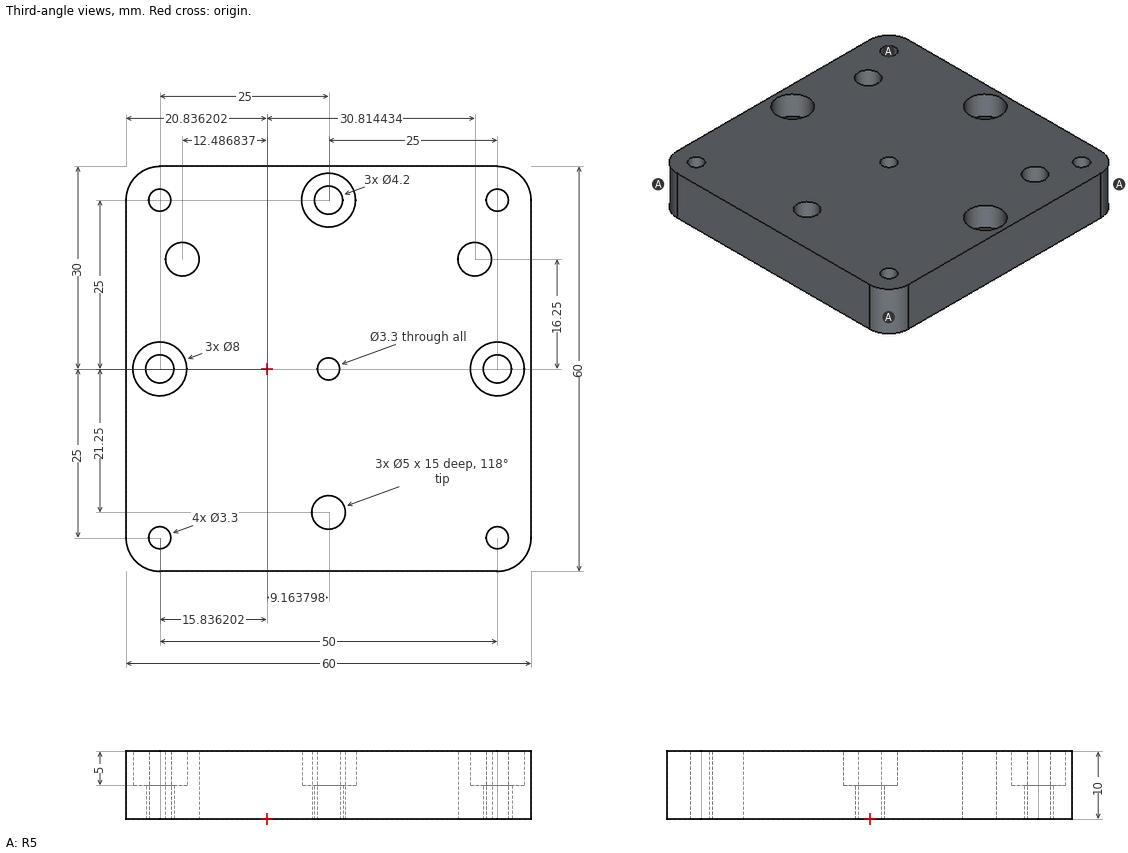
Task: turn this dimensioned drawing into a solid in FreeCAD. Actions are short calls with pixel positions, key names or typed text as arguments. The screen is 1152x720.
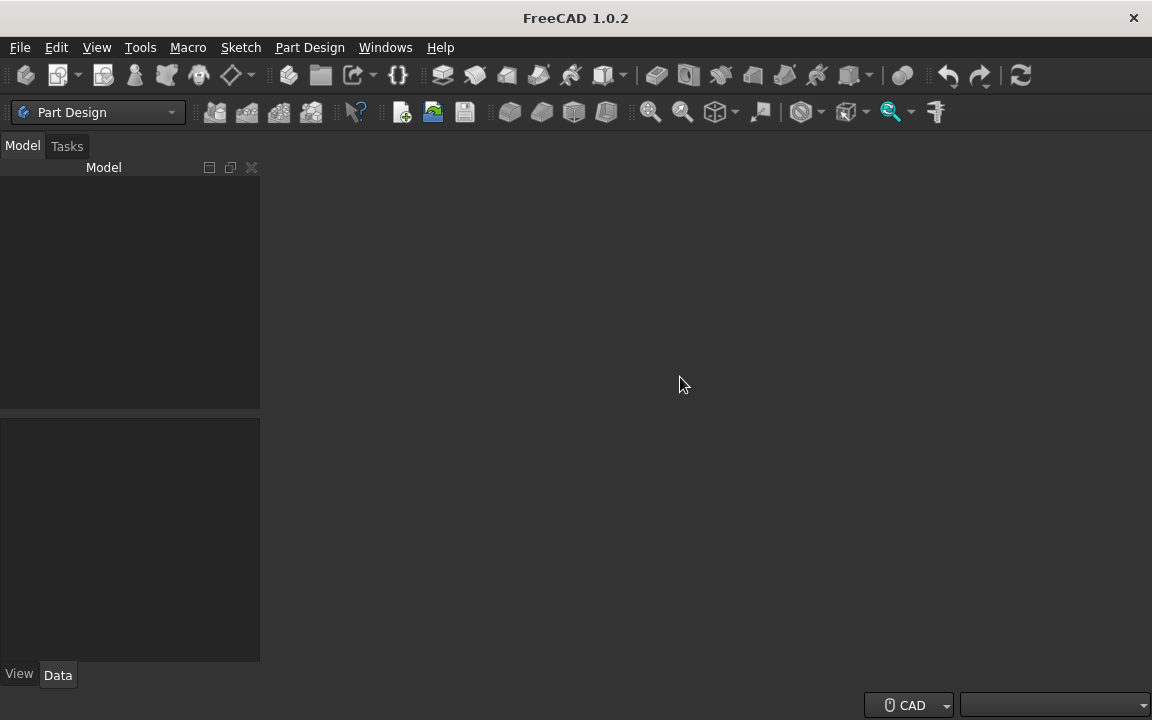
key(ctrl+n)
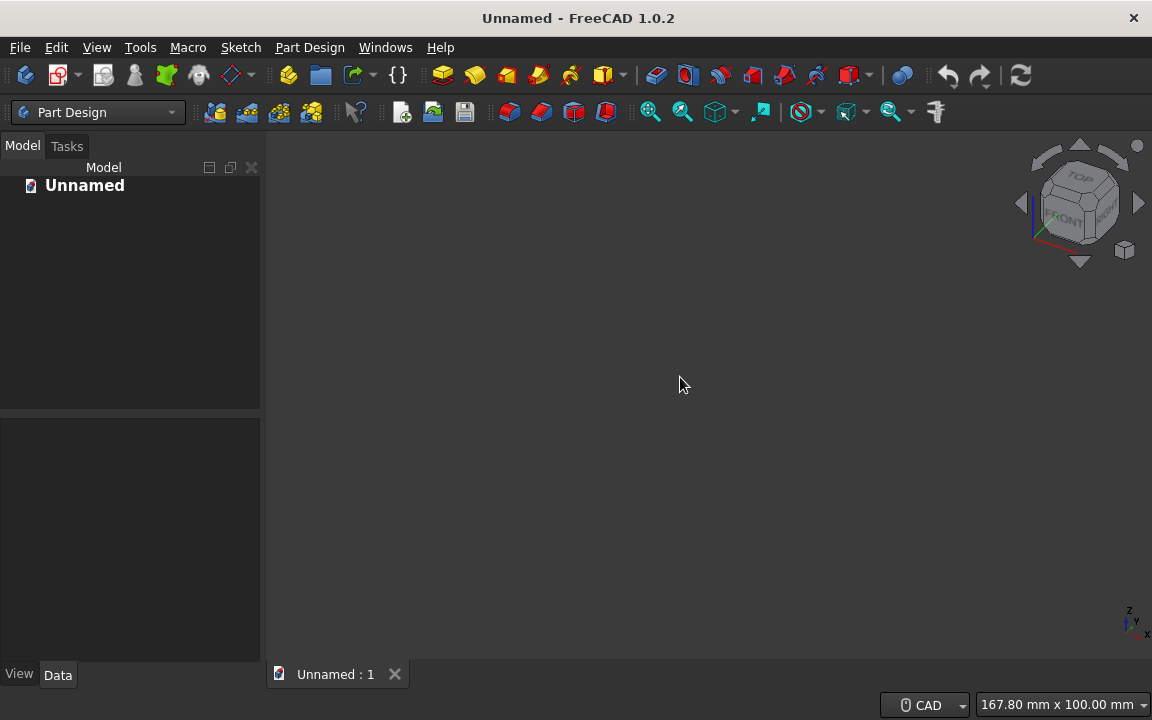
click(58, 76)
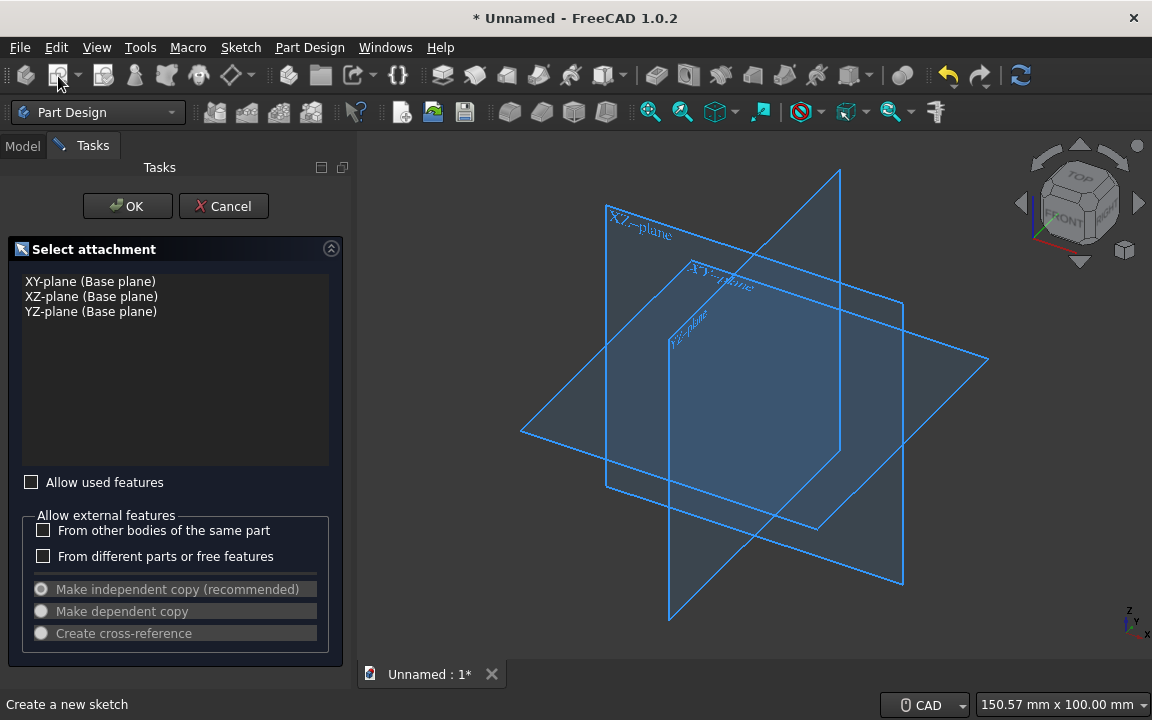
click(82, 282)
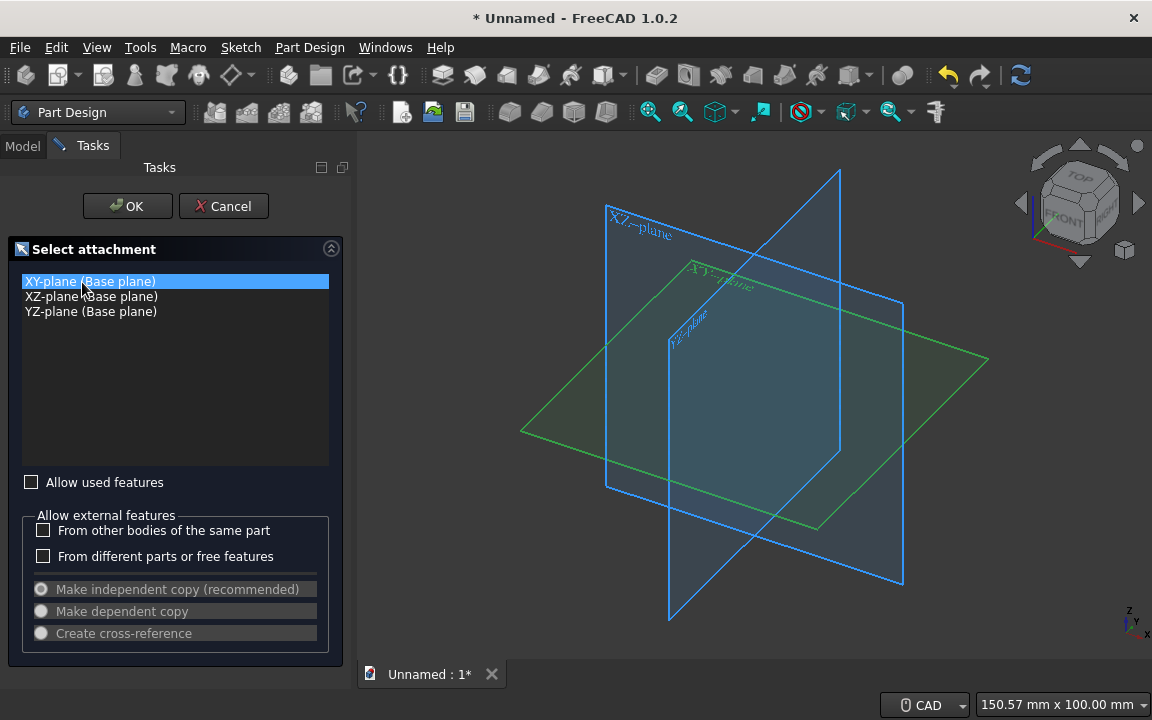
click(128, 206)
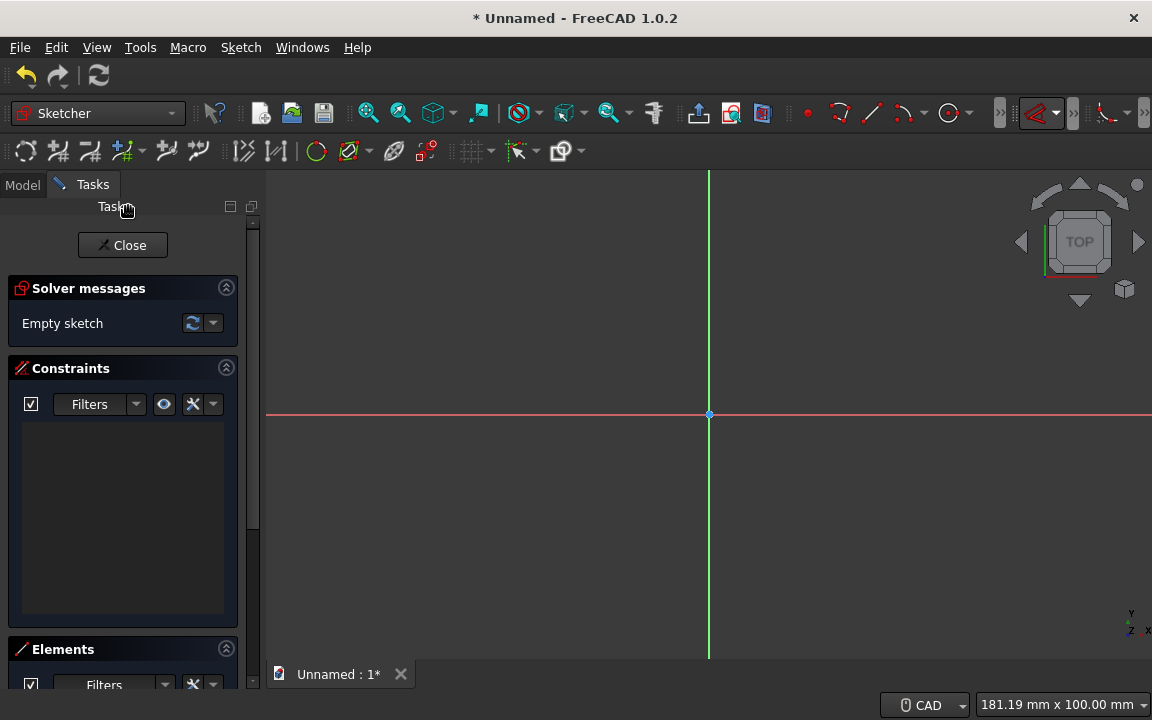
key(g)
key(r)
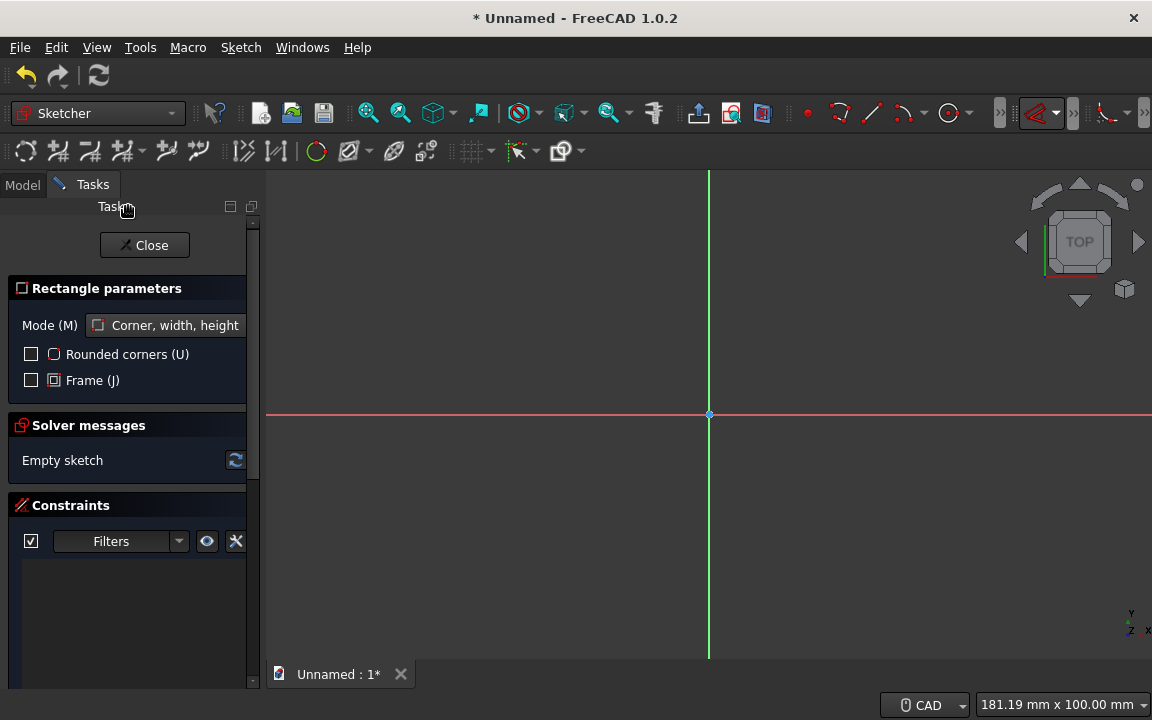
click(607, 268)
move(901, 561)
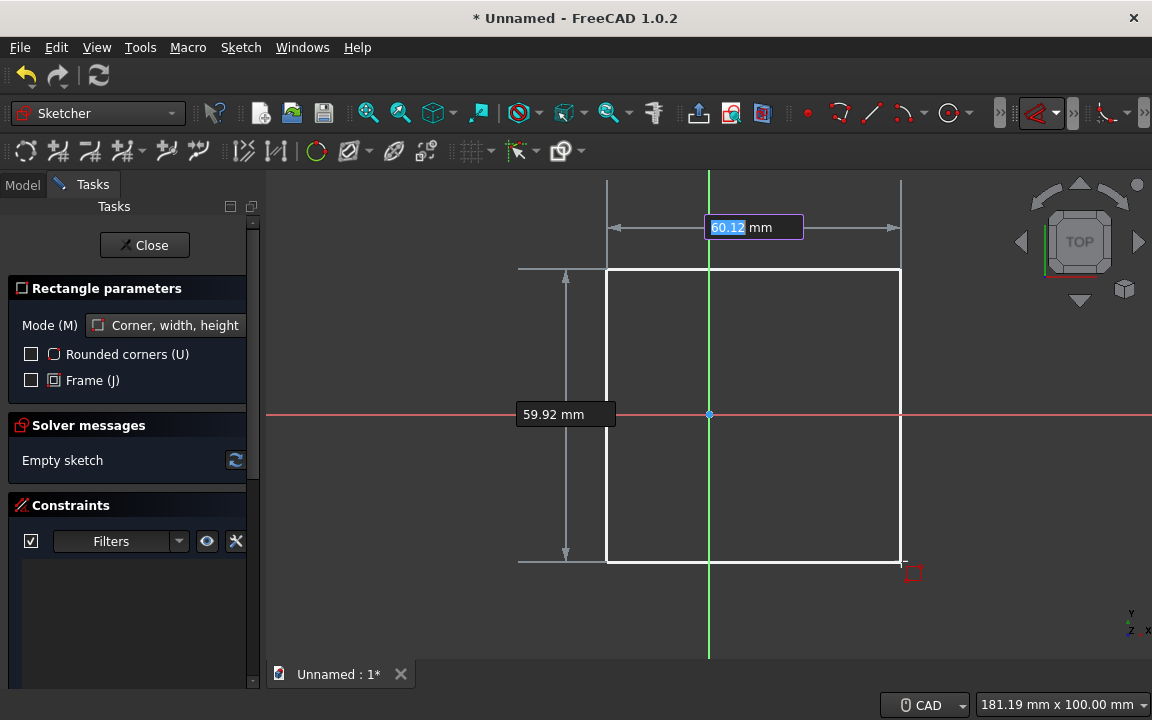
text(60)
key(Tab)
text(60)
key(Return)
key(Escape)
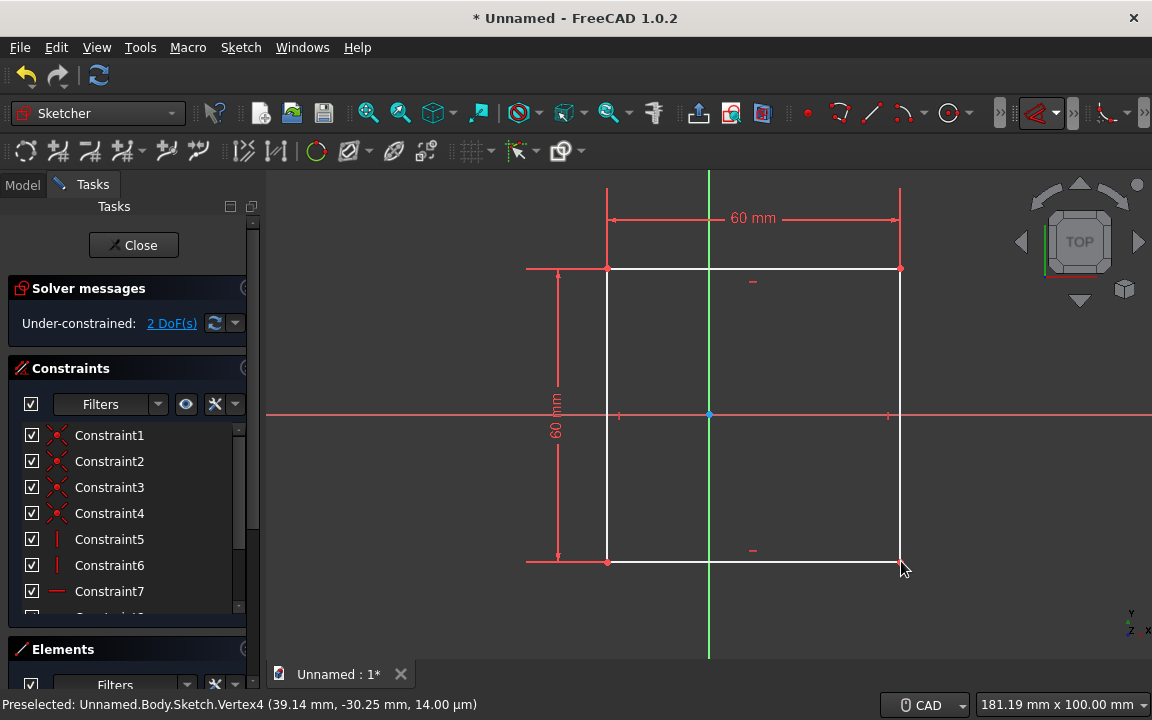
click(1036, 114)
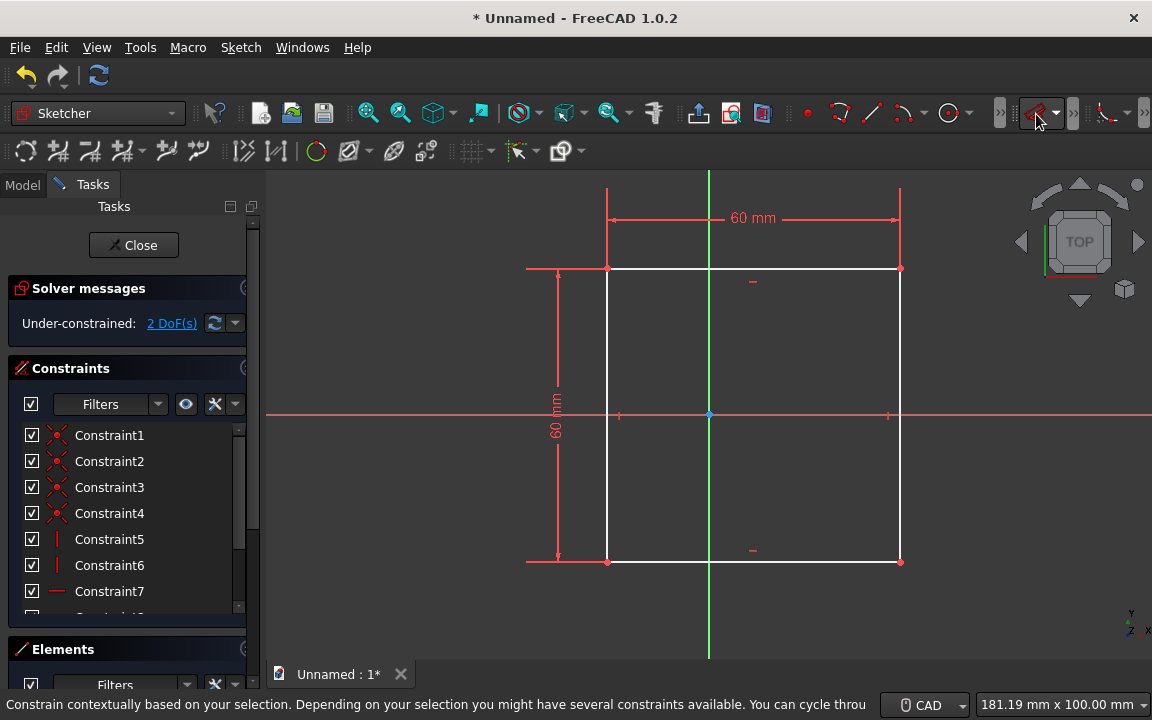
click(607, 269)
click(573, 342)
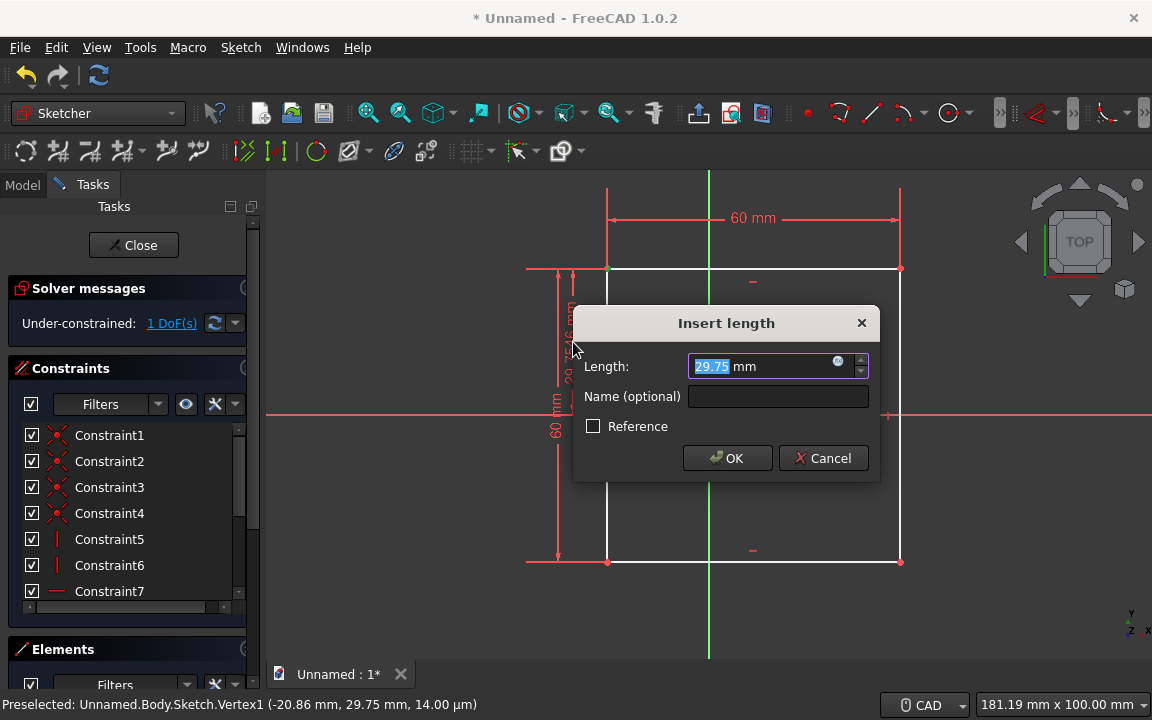
text(30)
key(Return)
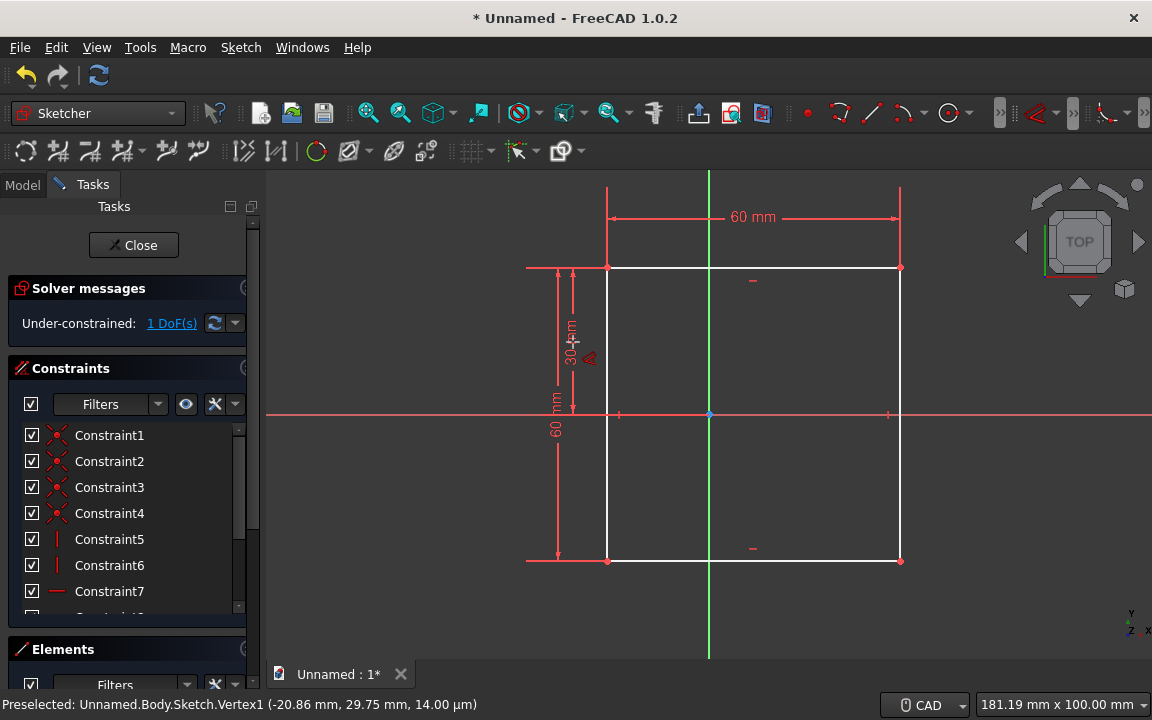
click(607, 268)
click(658, 234)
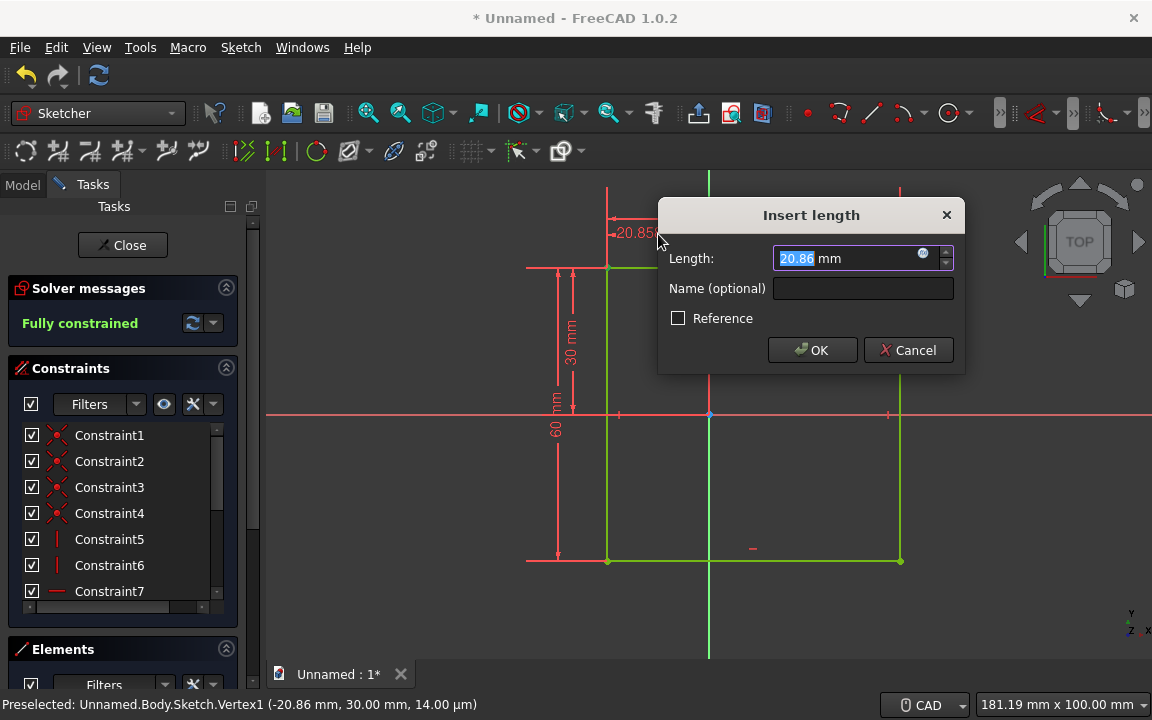
text(20.836202)
key(Return)
key(Escape)